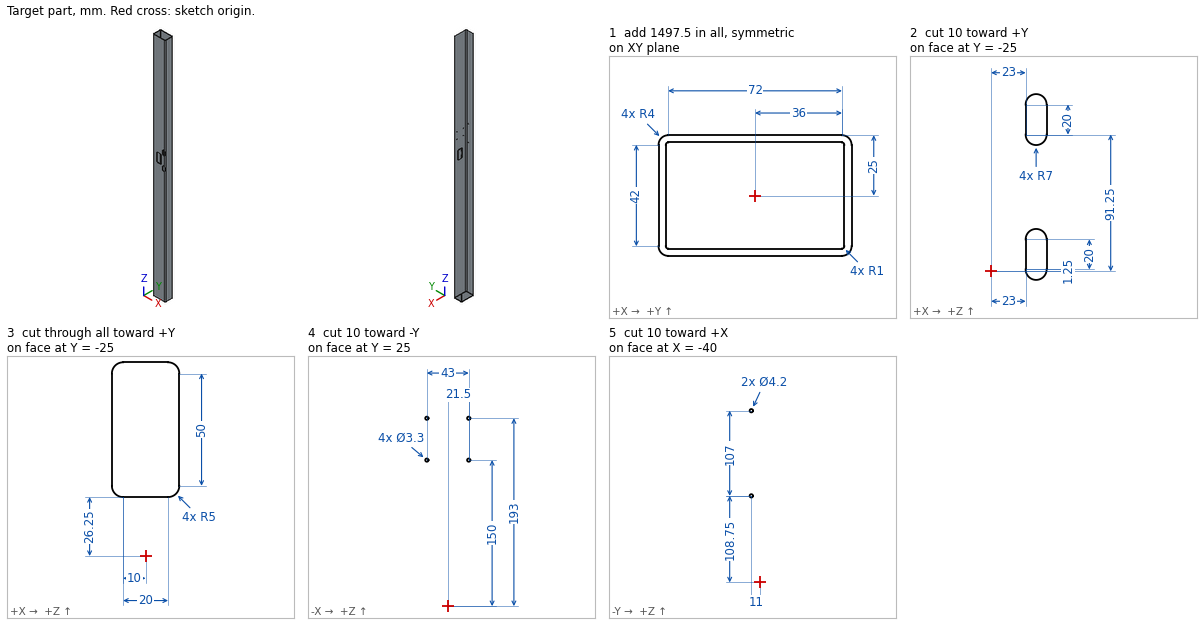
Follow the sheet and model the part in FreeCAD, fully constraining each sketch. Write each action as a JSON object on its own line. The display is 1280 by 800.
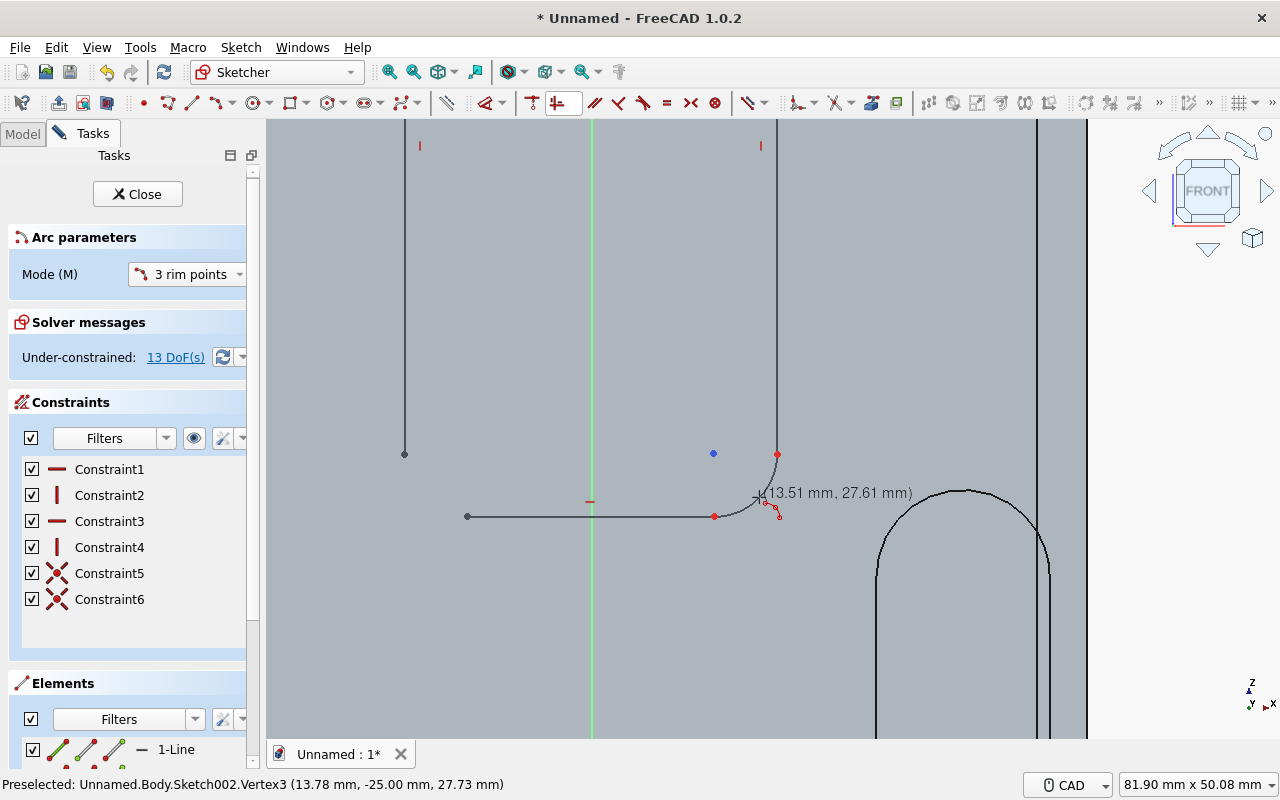
{"action": "scroll", "coordinate": [770, 501], "scroll_direction": "down", "scroll_amount": 5}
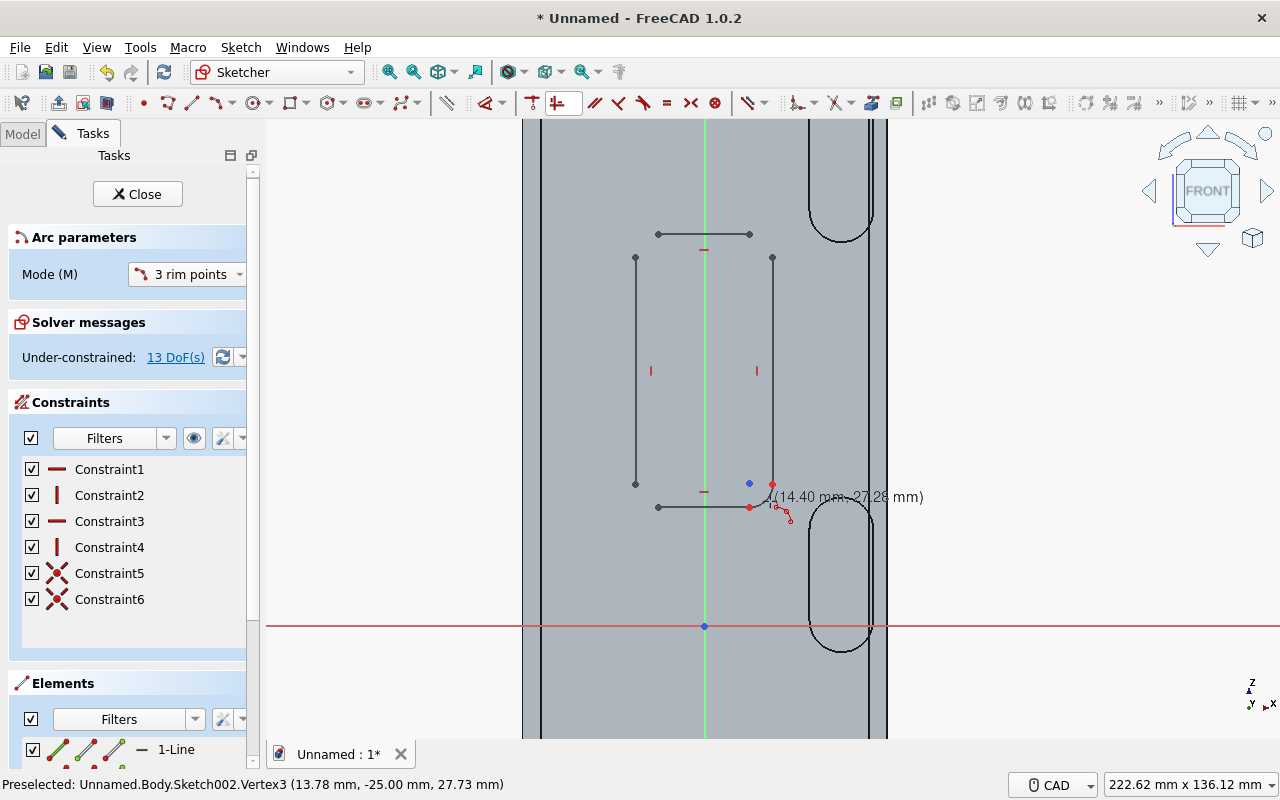
{"action": "left_click", "coordinate": [773, 257]}
{"action": "left_click", "coordinate": [750, 234]}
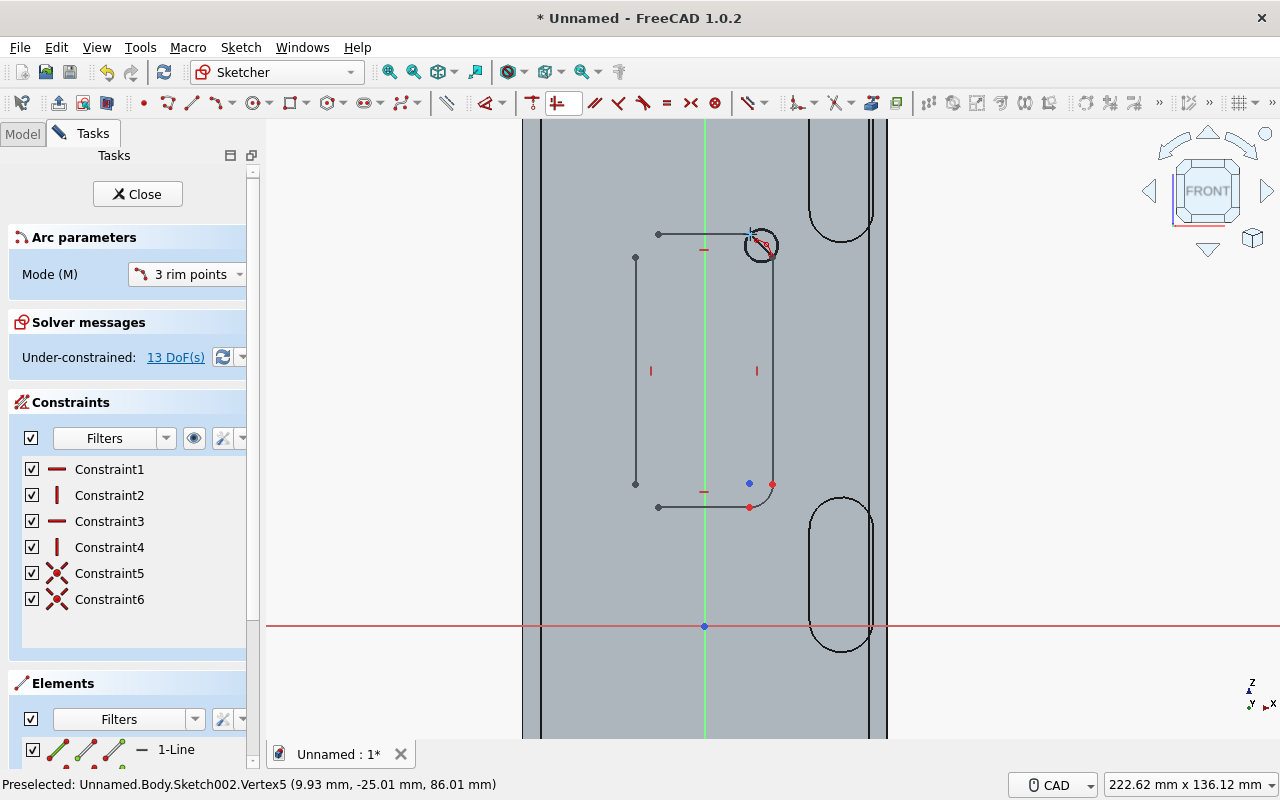
{"action": "scroll", "coordinate": [766, 240], "scroll_direction": "up", "scroll_amount": 5}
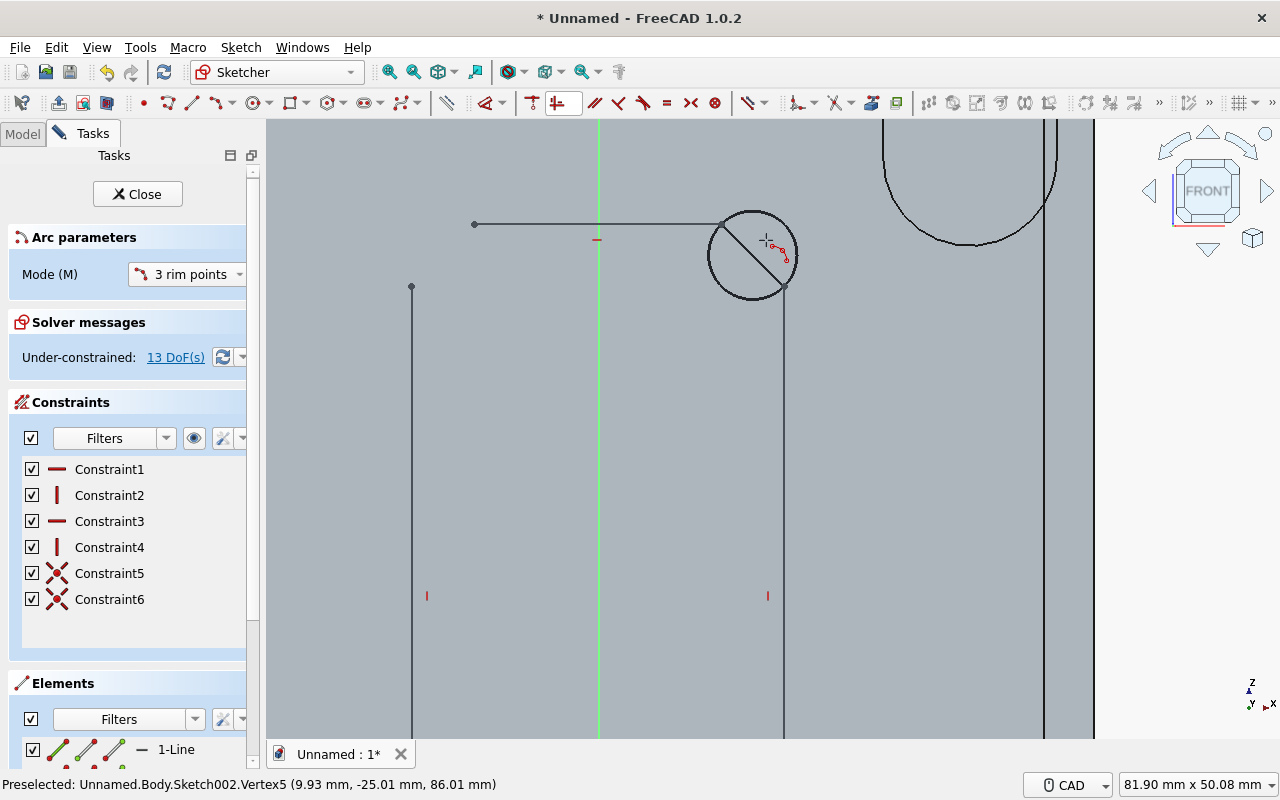
{"action": "left_click", "coordinate": [766, 239]}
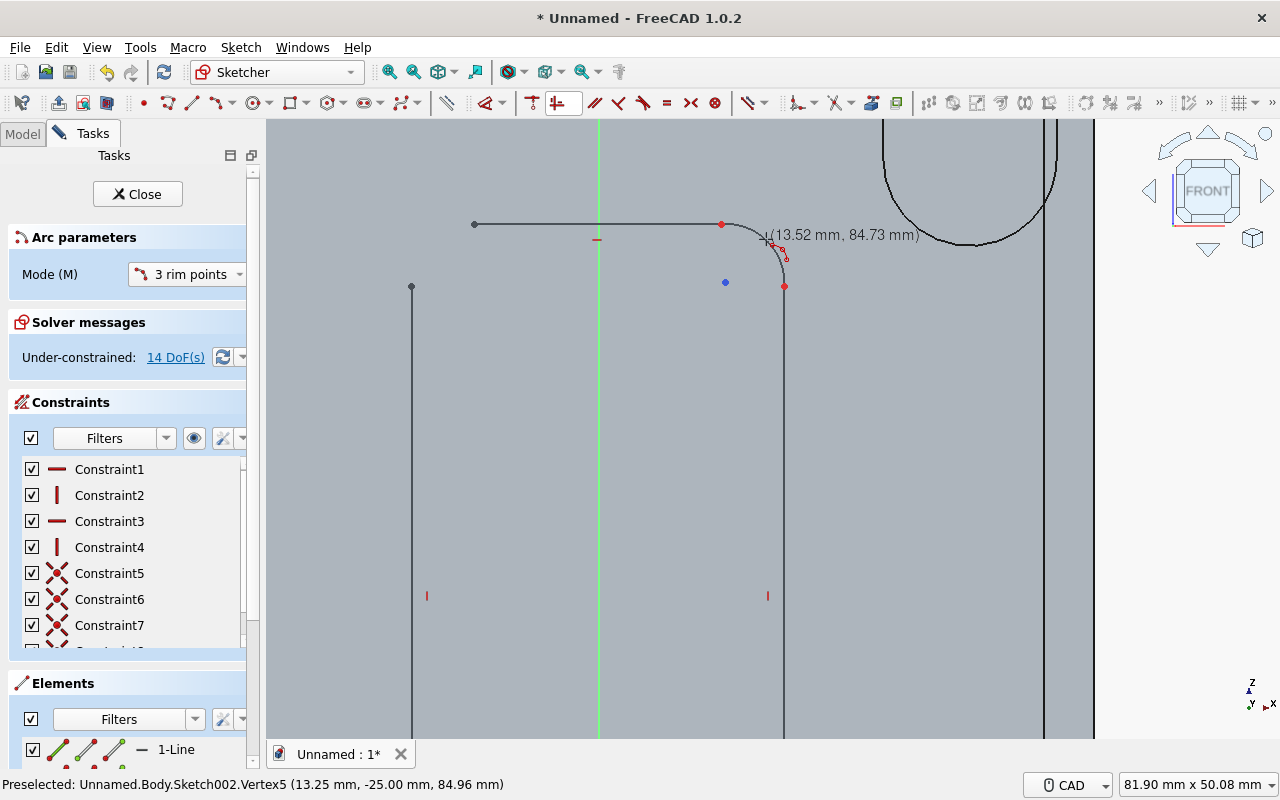
{"action": "left_click", "coordinate": [474, 224]}
{"action": "left_click", "coordinate": [412, 287]}
{"action": "left_click", "coordinate": [431, 239]}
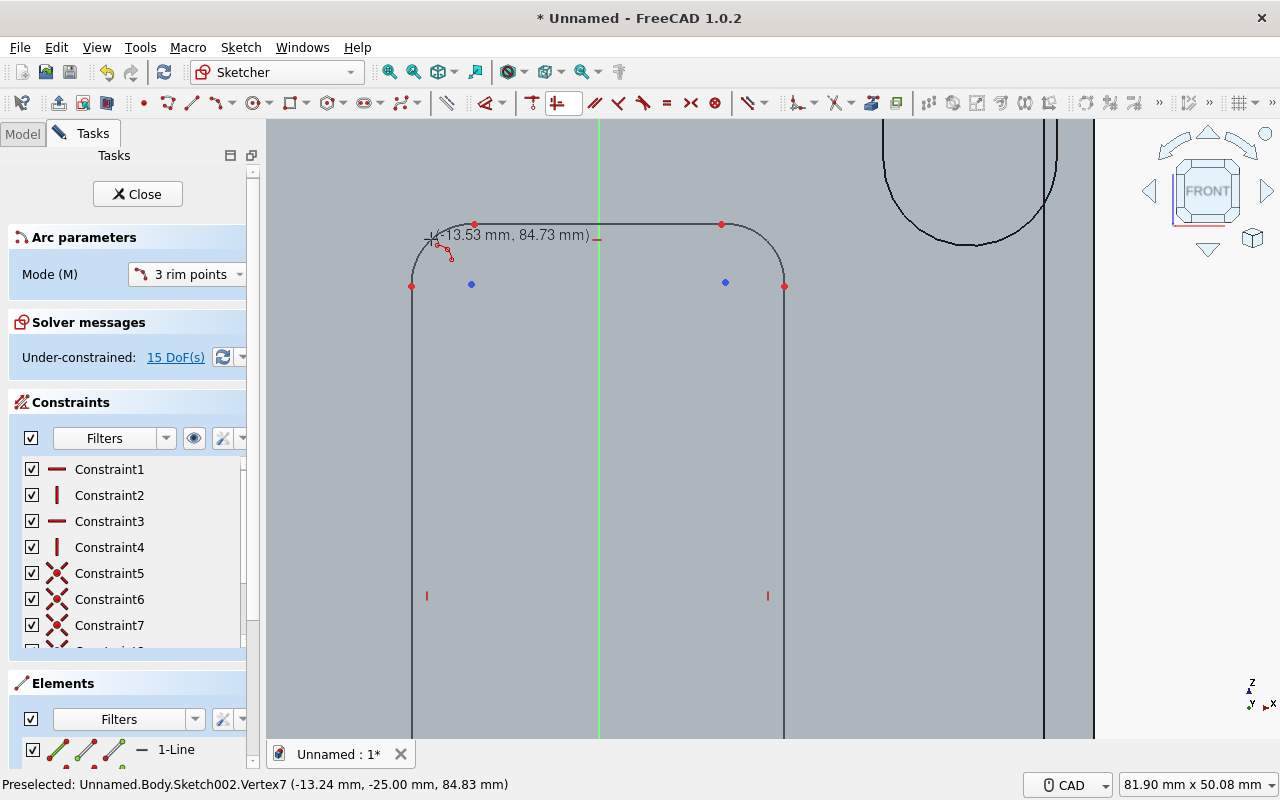
{"action": "scroll", "coordinate": [766, 239], "scroll_direction": "down", "scroll_amount": 5}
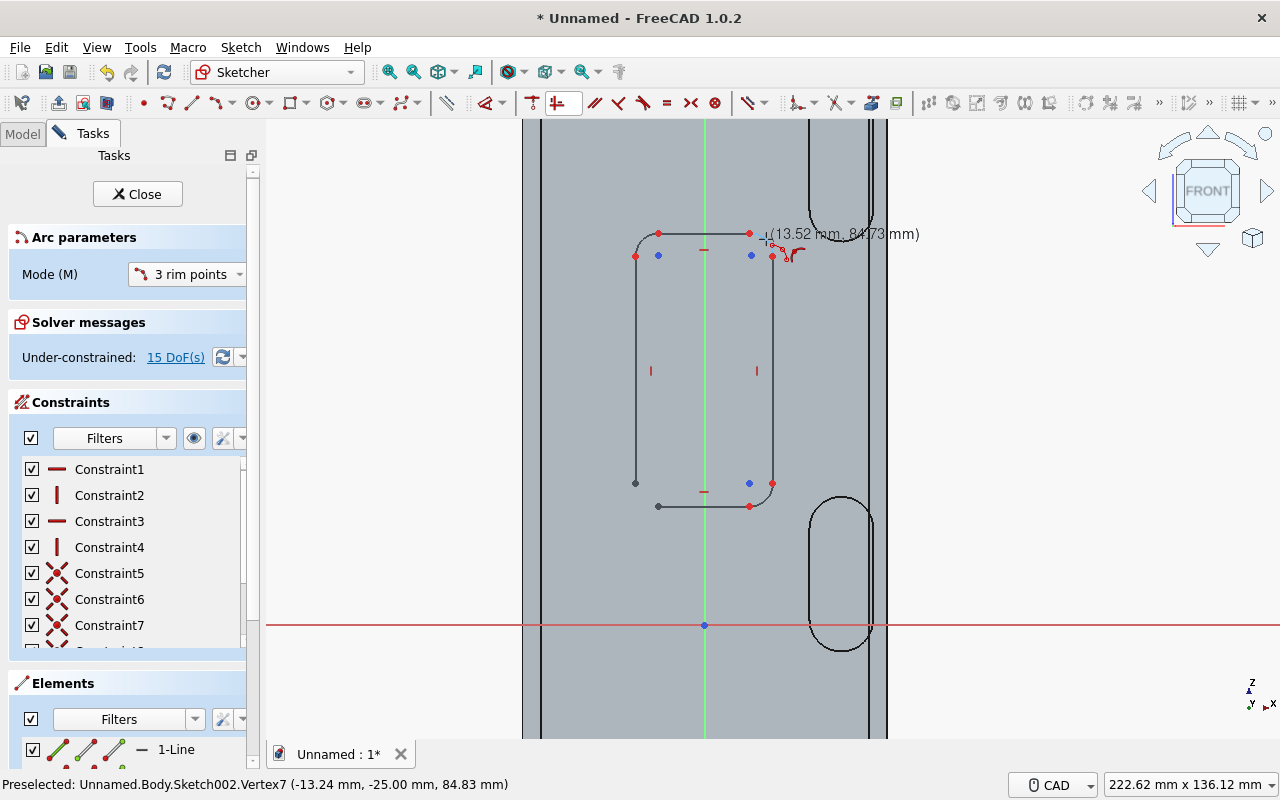
{"action": "left_click", "coordinate": [636, 484]}
{"action": "left_click", "coordinate": [659, 507]}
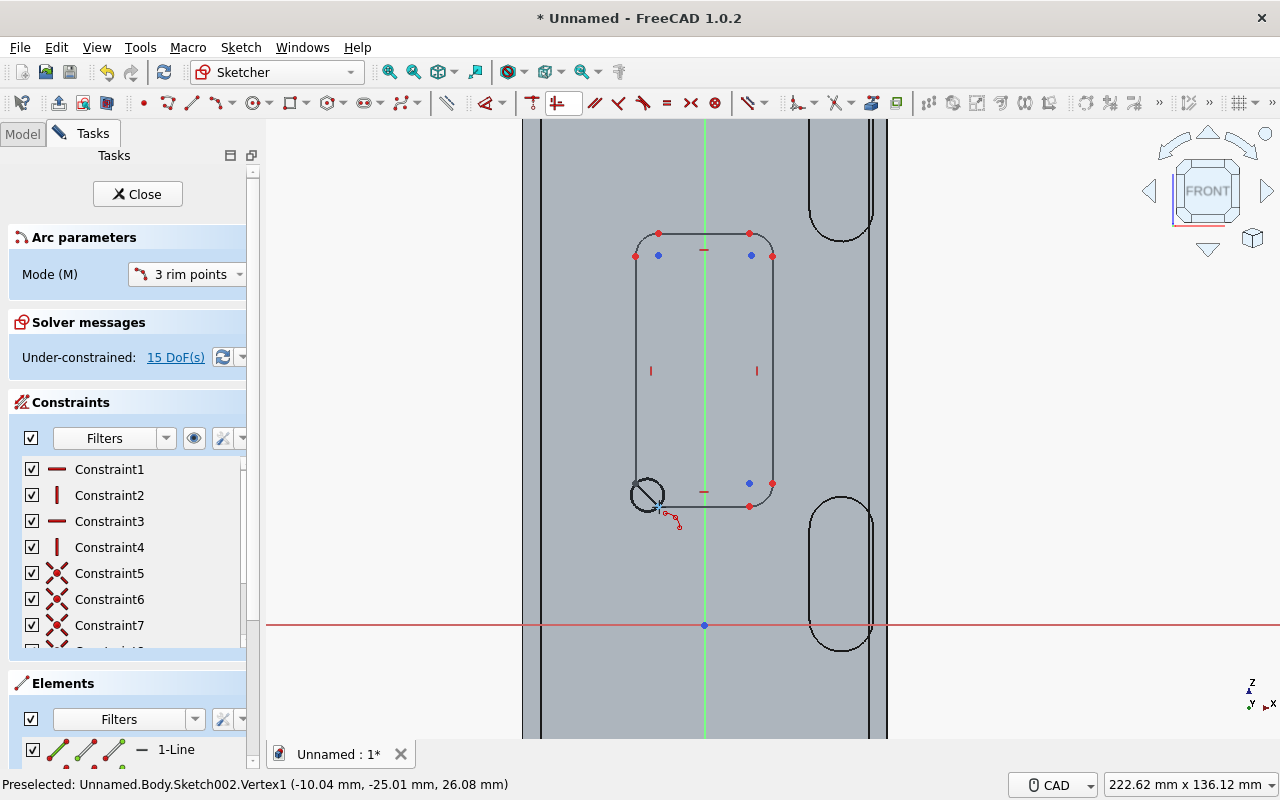
{"action": "scroll", "coordinate": [643, 499], "scroll_direction": "up", "scroll_amount": 5}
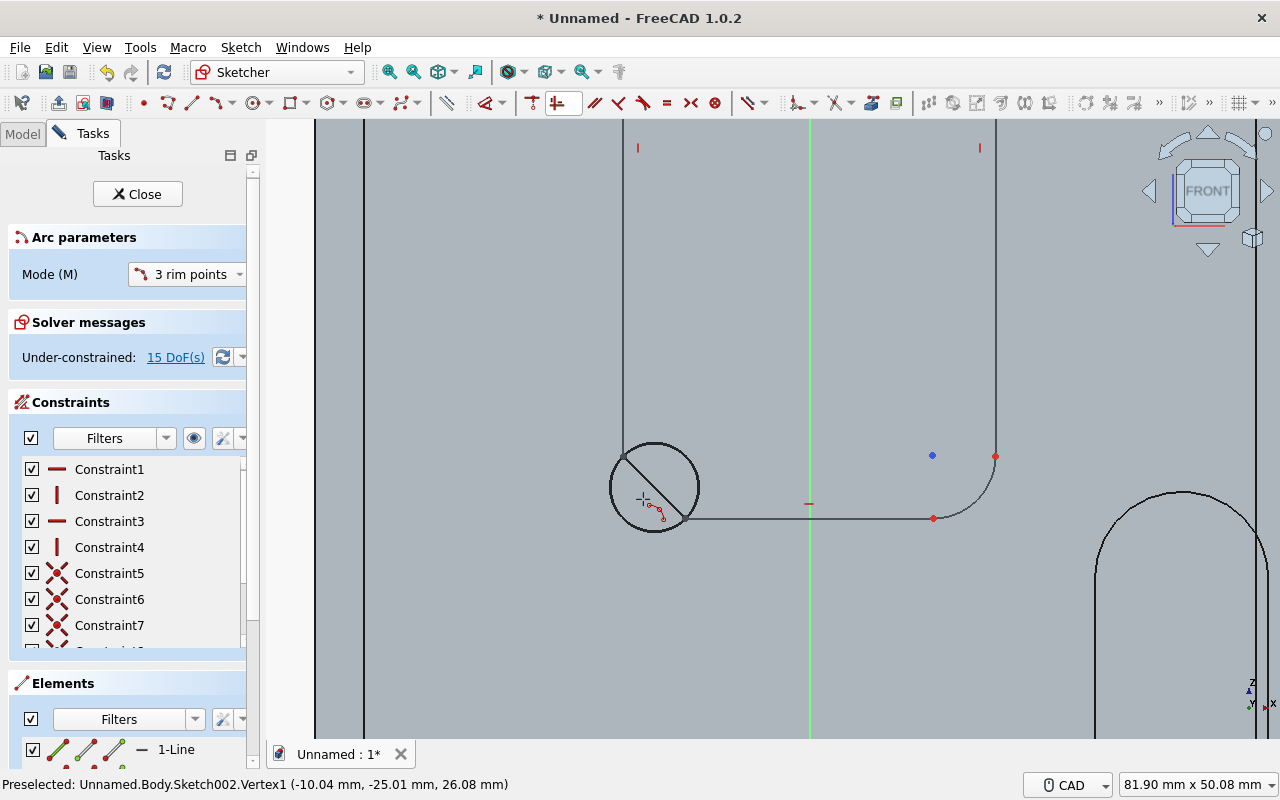
{"action": "left_click", "coordinate": [643, 498]}
{"action": "key", "text": "Escape"}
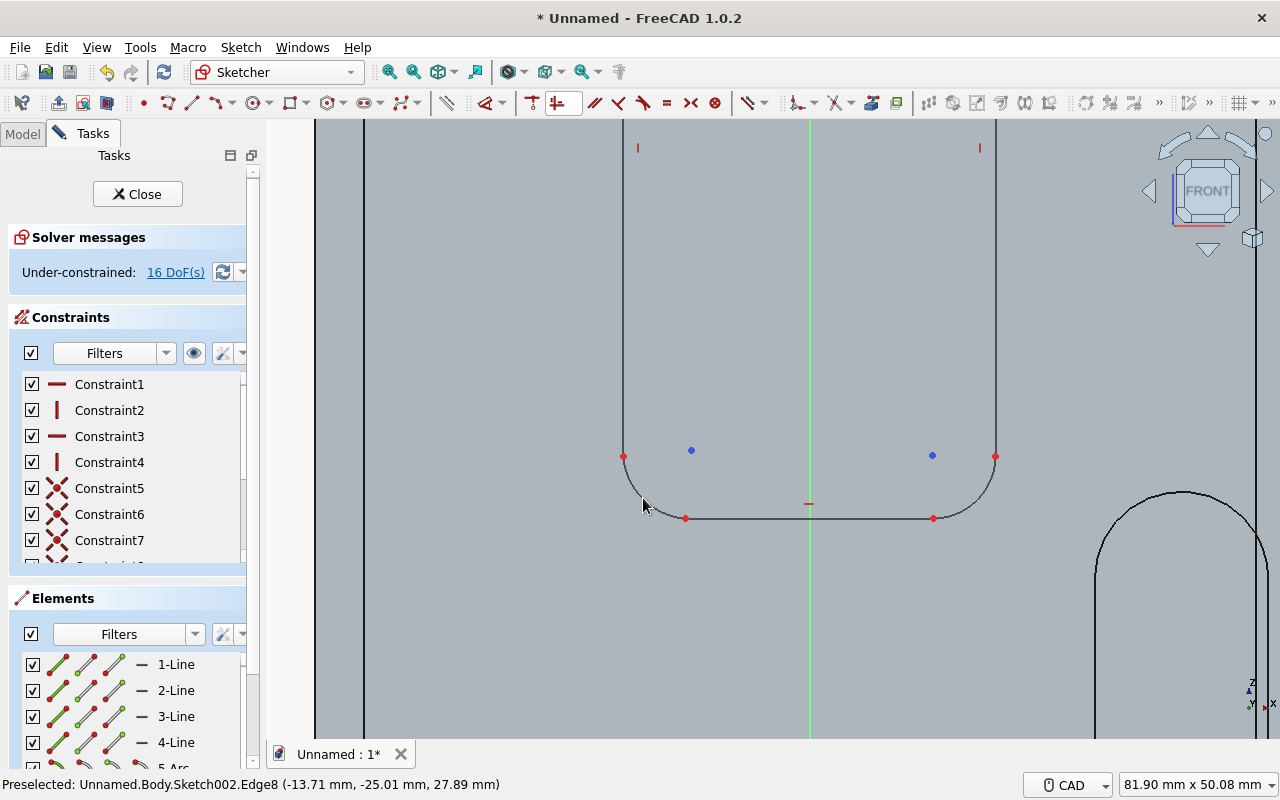
{"action": "left_click", "coordinate": [760, 519]}